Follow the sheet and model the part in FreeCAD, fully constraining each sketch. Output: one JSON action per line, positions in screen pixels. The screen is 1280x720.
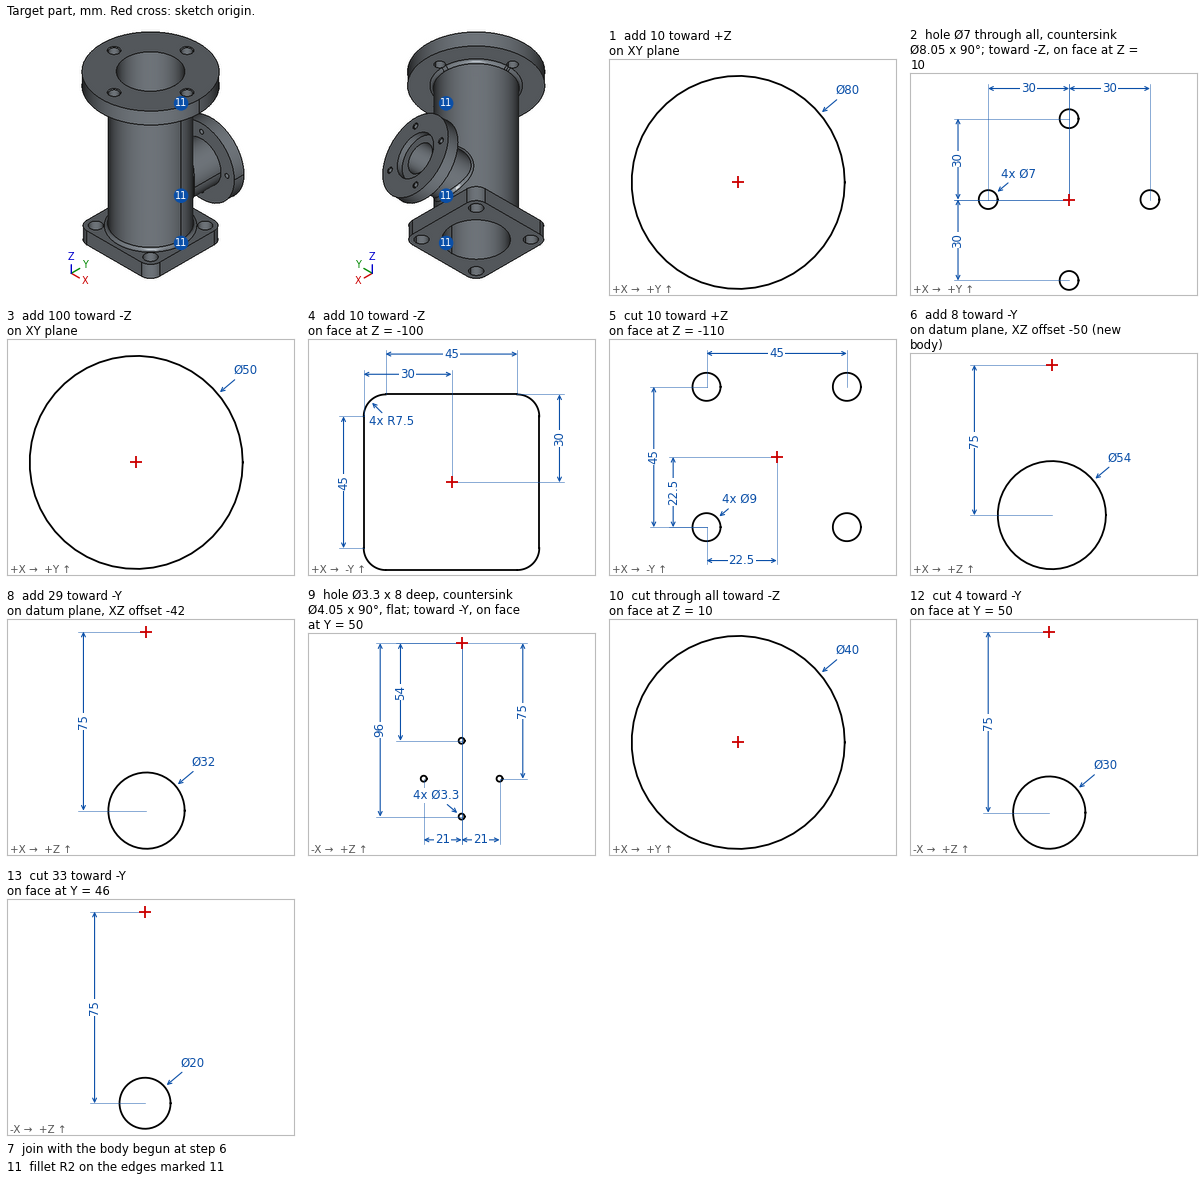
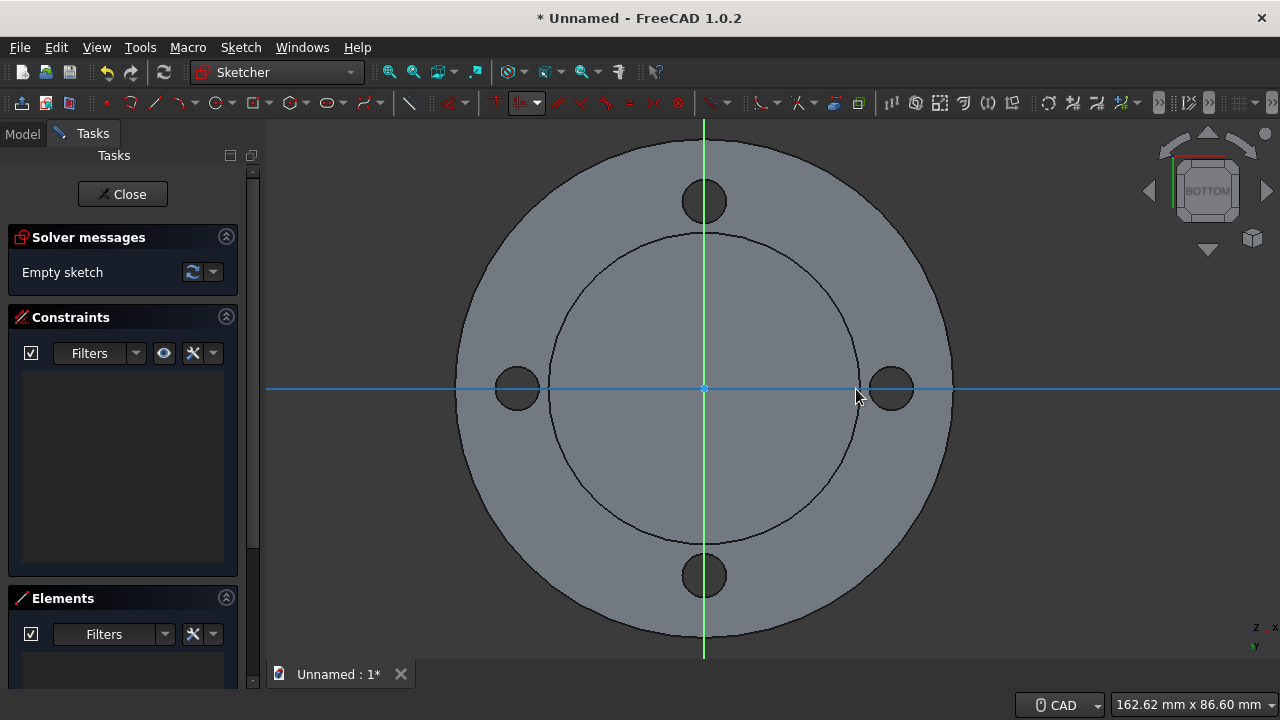
{"action": "left_click", "coordinate": [156, 104]}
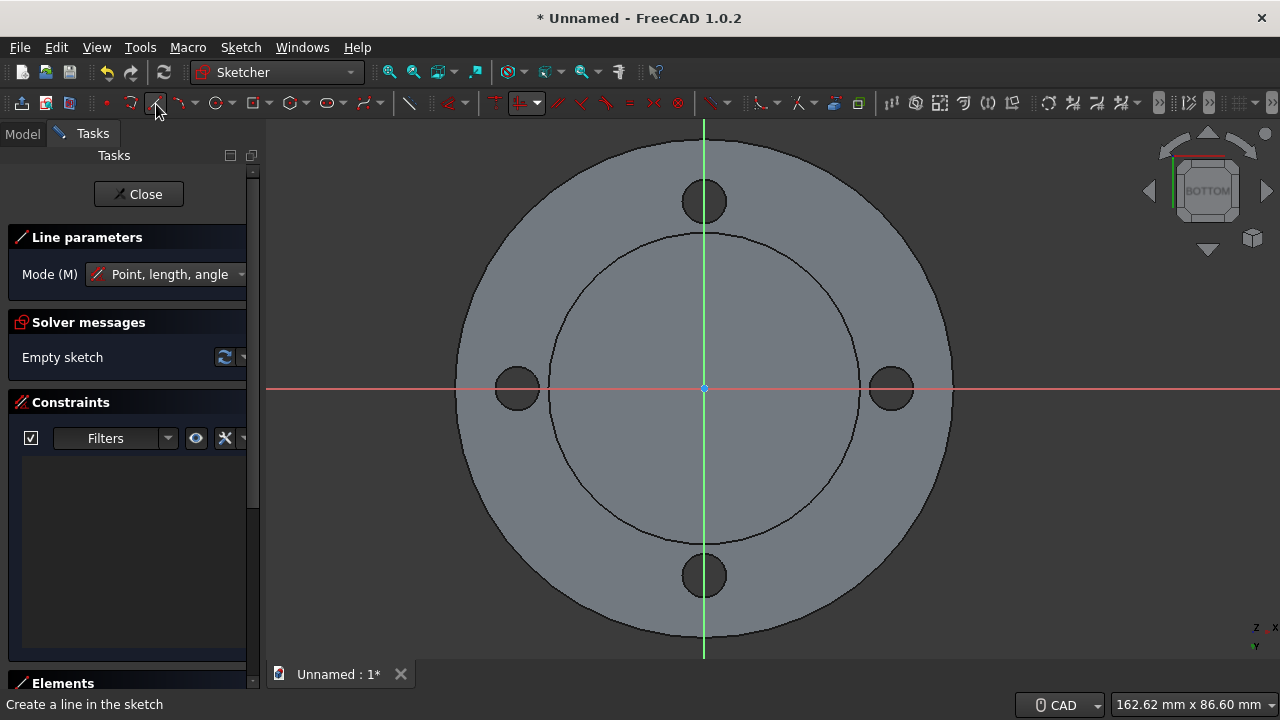
{"action": "left_click", "coordinate": [845, 202]}
{"action": "left_click", "coordinate": [564, 202]}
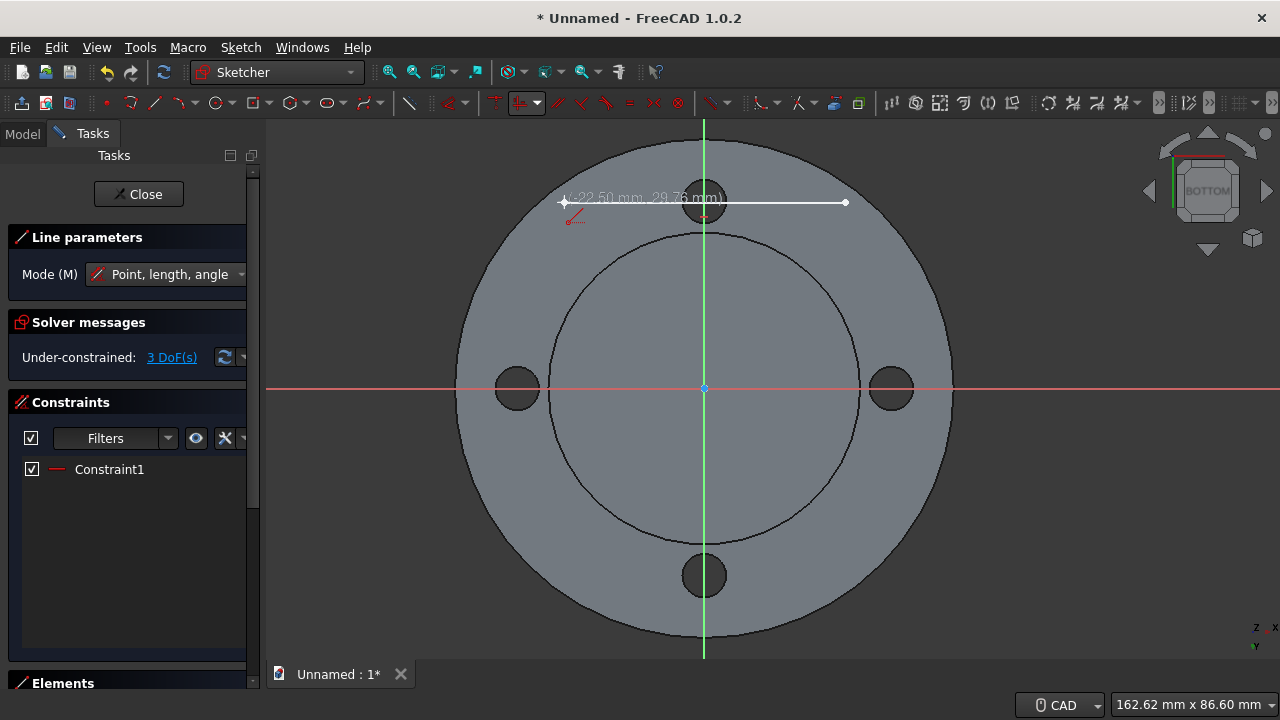
{"action": "left_click", "coordinate": [517, 248]}
{"action": "left_click", "coordinate": [517, 529]}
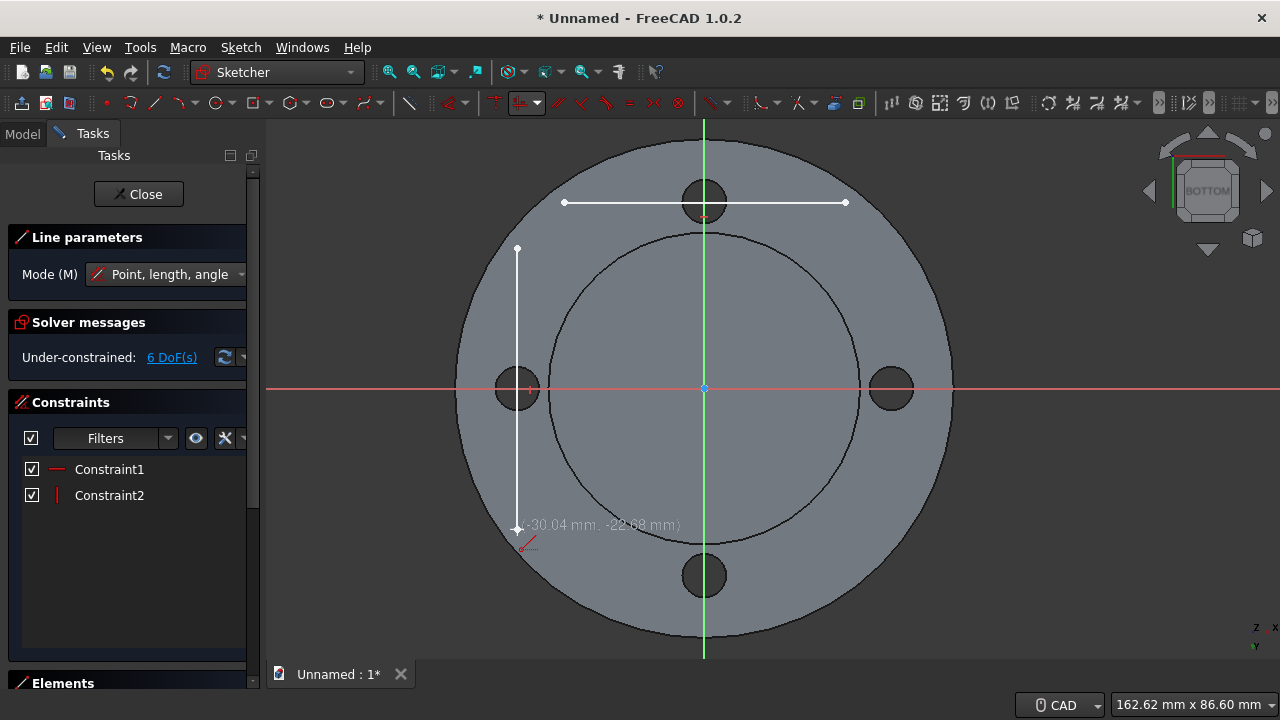
{"action": "left_click", "coordinate": [564, 576]}
{"action": "left_click", "coordinate": [845, 576]}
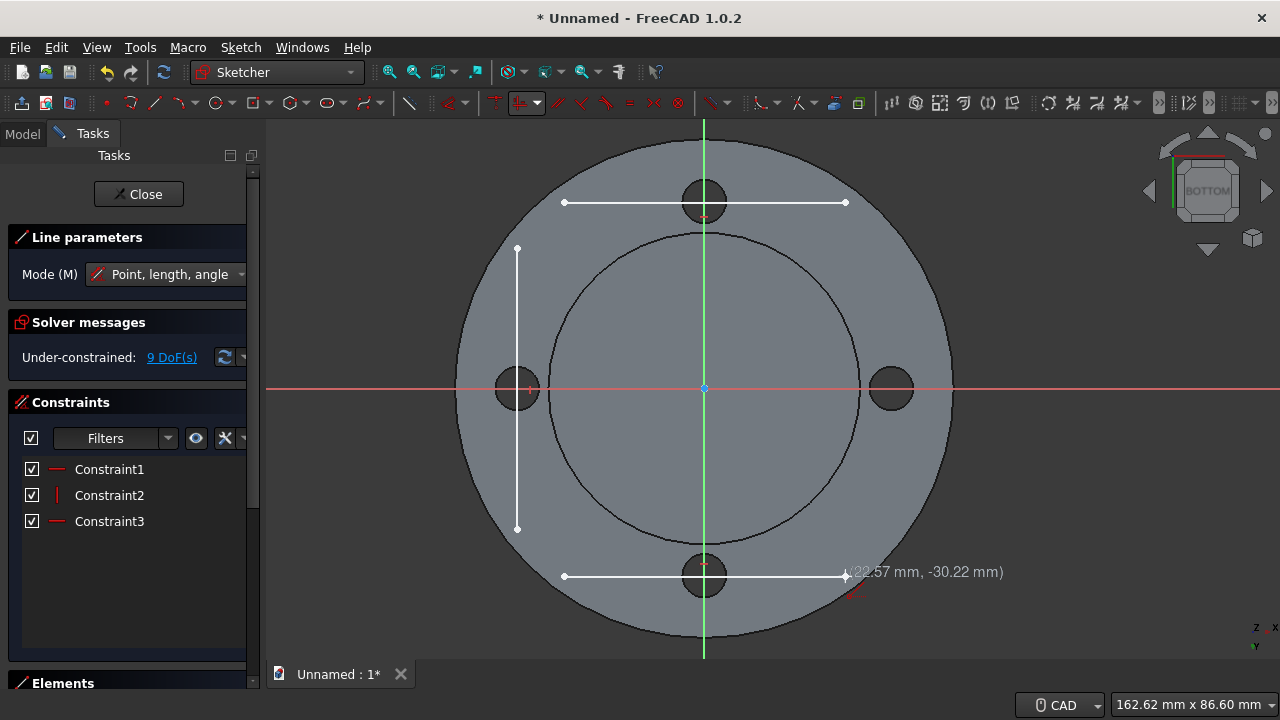
{"action": "left_click", "coordinate": [891, 529]}
{"action": "left_click", "coordinate": [891, 248]}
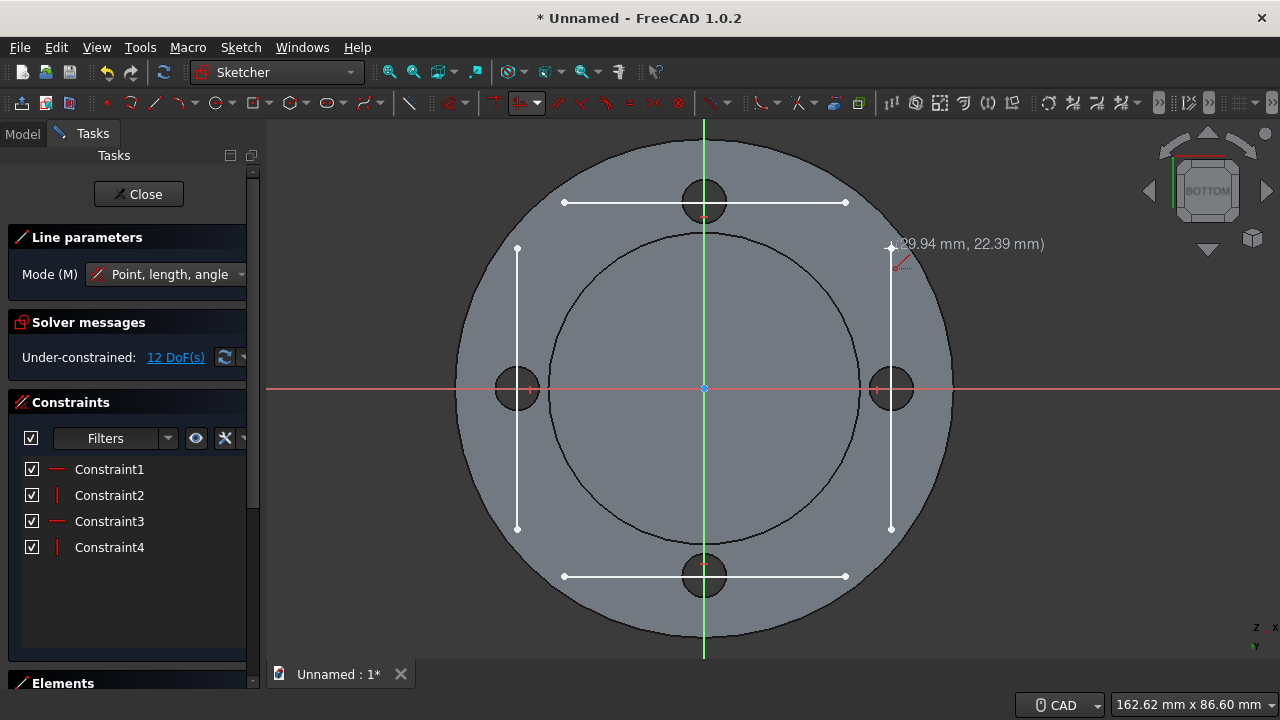
{"action": "left_click", "coordinate": [180, 104]}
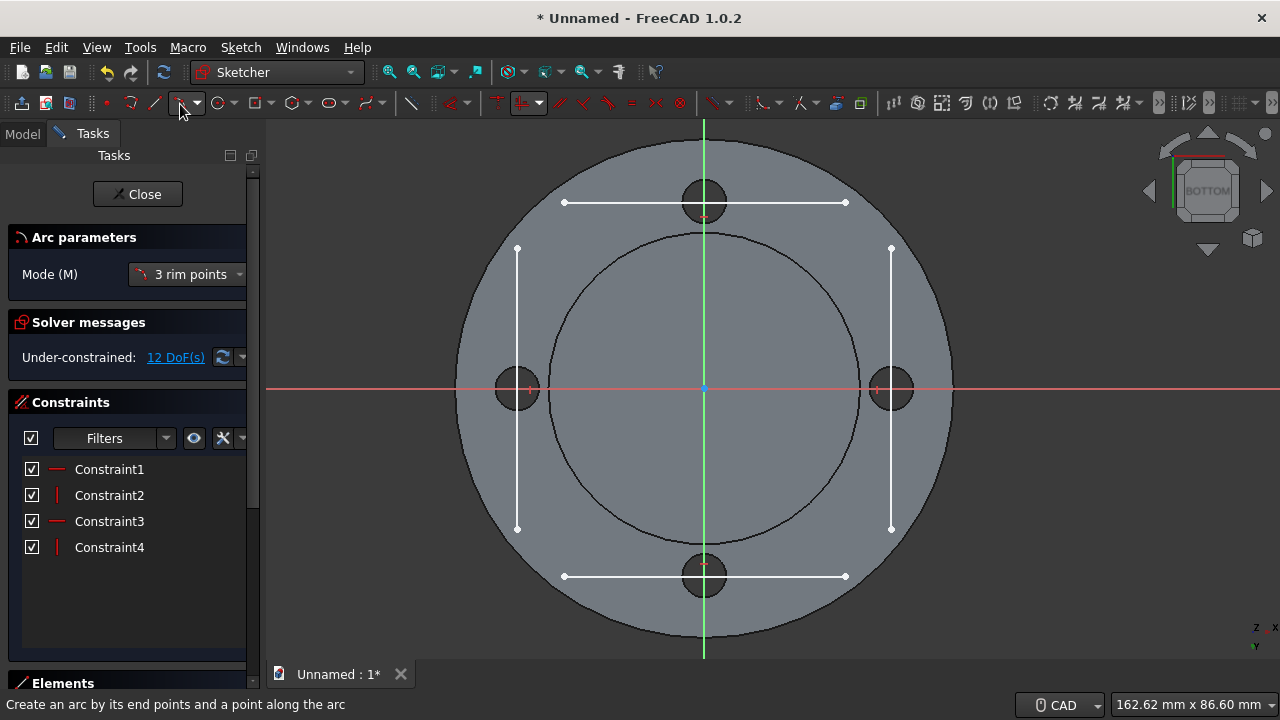
{"action": "left_click", "coordinate": [564, 203]}
{"action": "left_click", "coordinate": [517, 249]}
{"action": "left_click", "coordinate": [531, 215]}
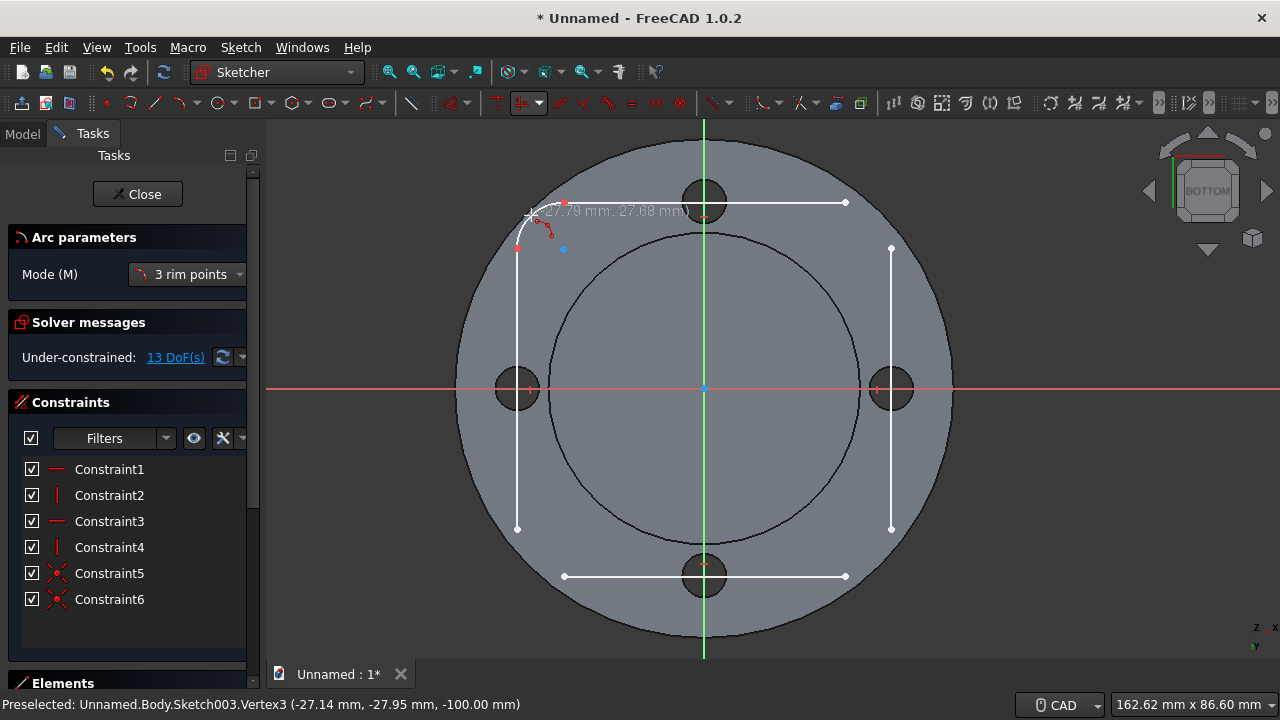
{"action": "left_click", "coordinate": [517, 530]}
{"action": "left_click", "coordinate": [564, 577]}
{"action": "left_click", "coordinate": [531, 562]}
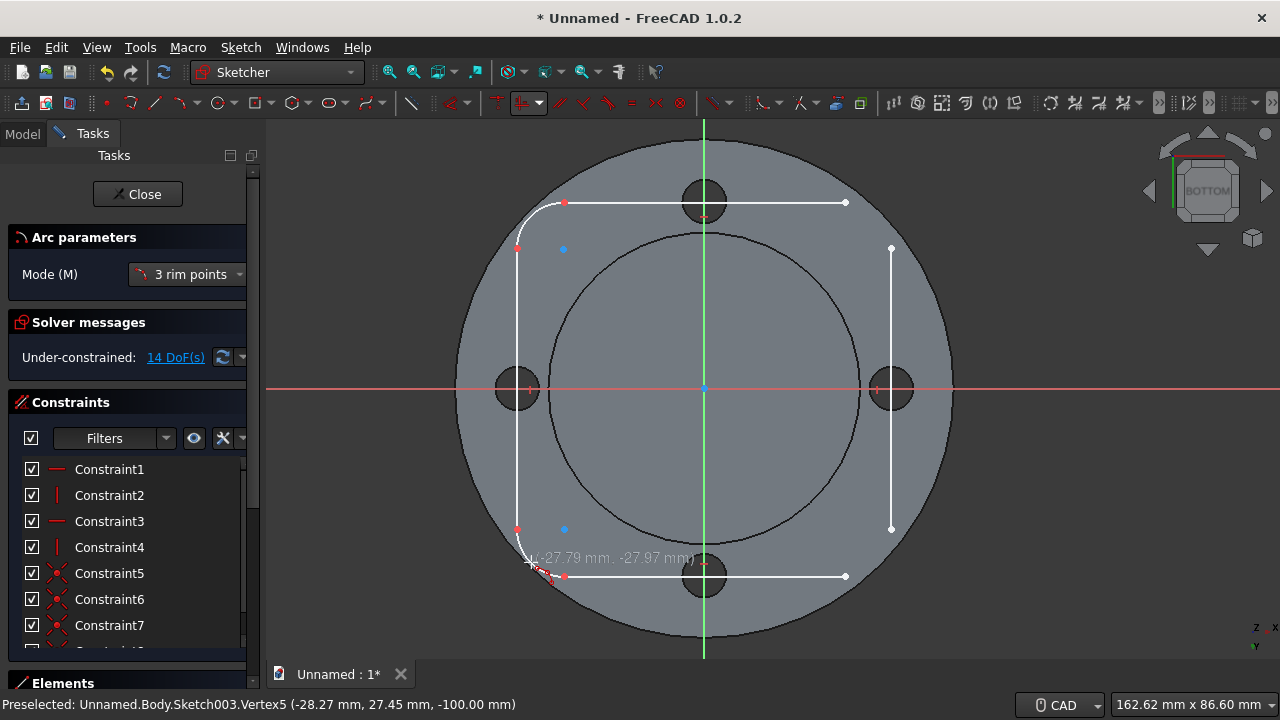
{"action": "left_click", "coordinate": [845, 577]}
{"action": "left_click", "coordinate": [891, 530]}
{"action": "left_click", "coordinate": [878, 562]}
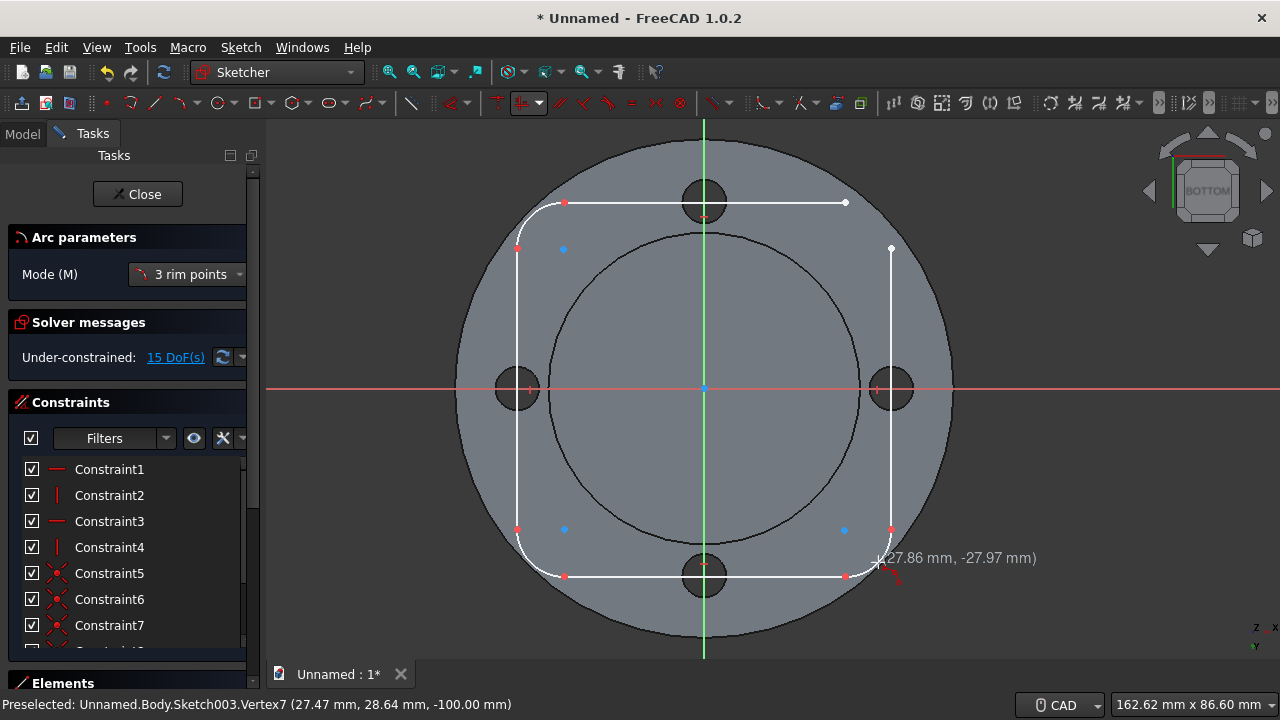
{"action": "left_click", "coordinate": [891, 249]}
{"action": "left_click", "coordinate": [845, 203]}
{"action": "left_click", "coordinate": [878, 215]}
{"action": "key", "text": "Escape"}